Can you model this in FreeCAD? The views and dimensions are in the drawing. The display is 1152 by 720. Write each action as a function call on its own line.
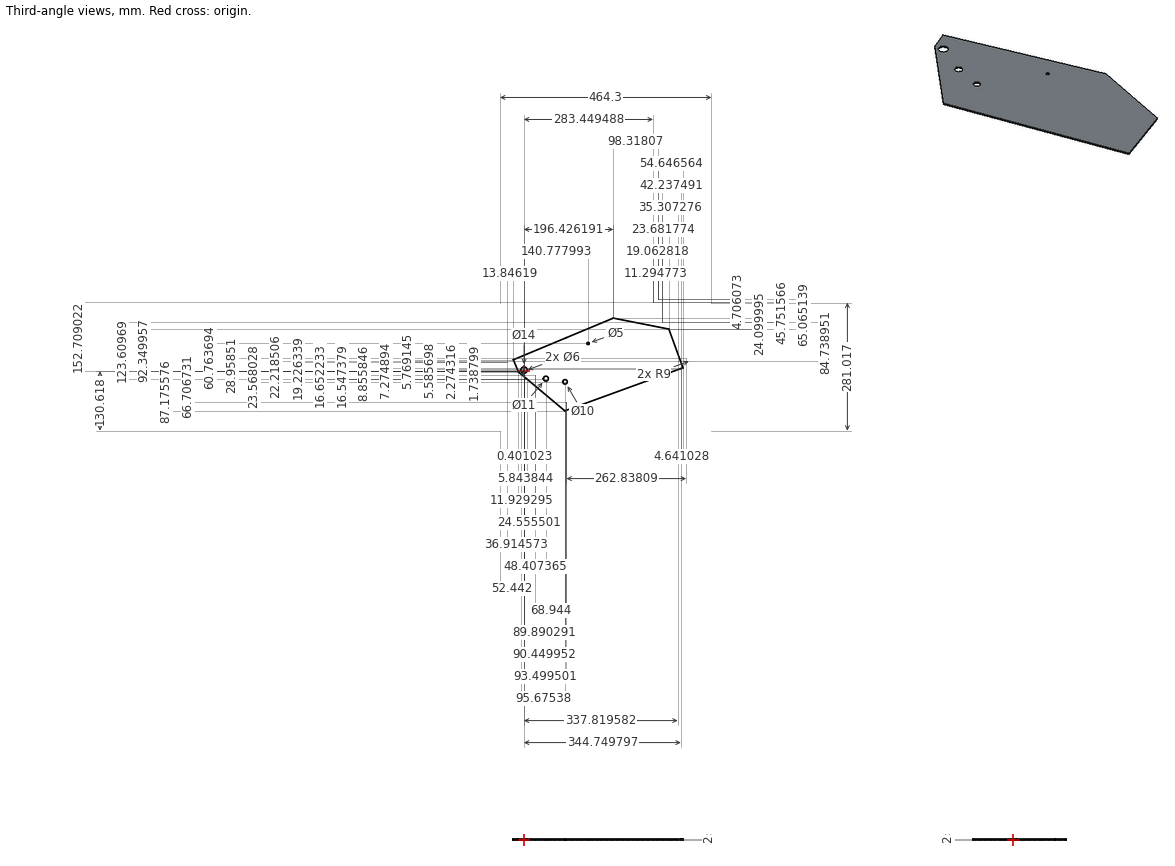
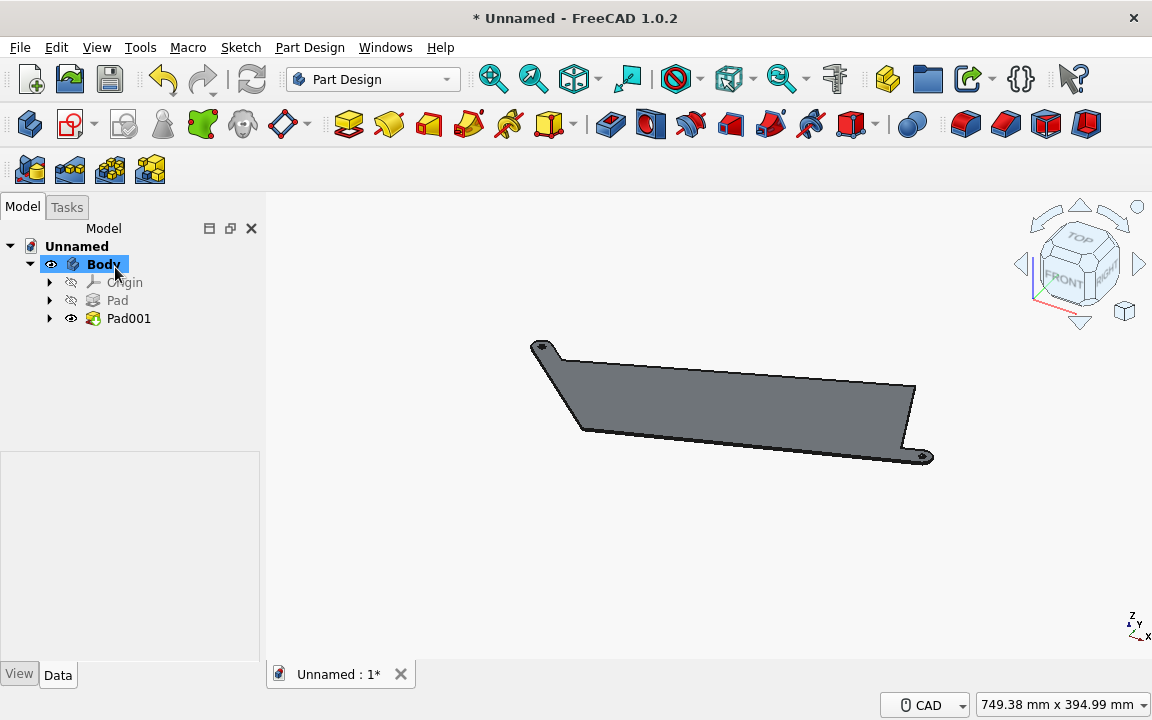
key(5)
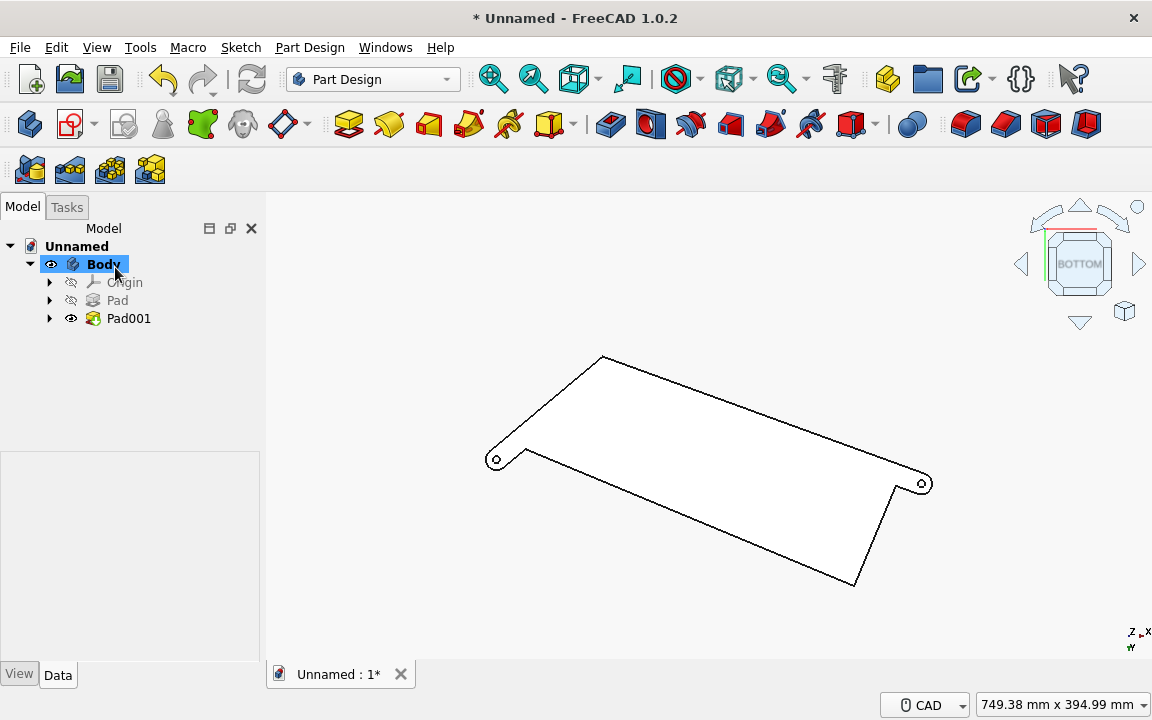
click(645, 438)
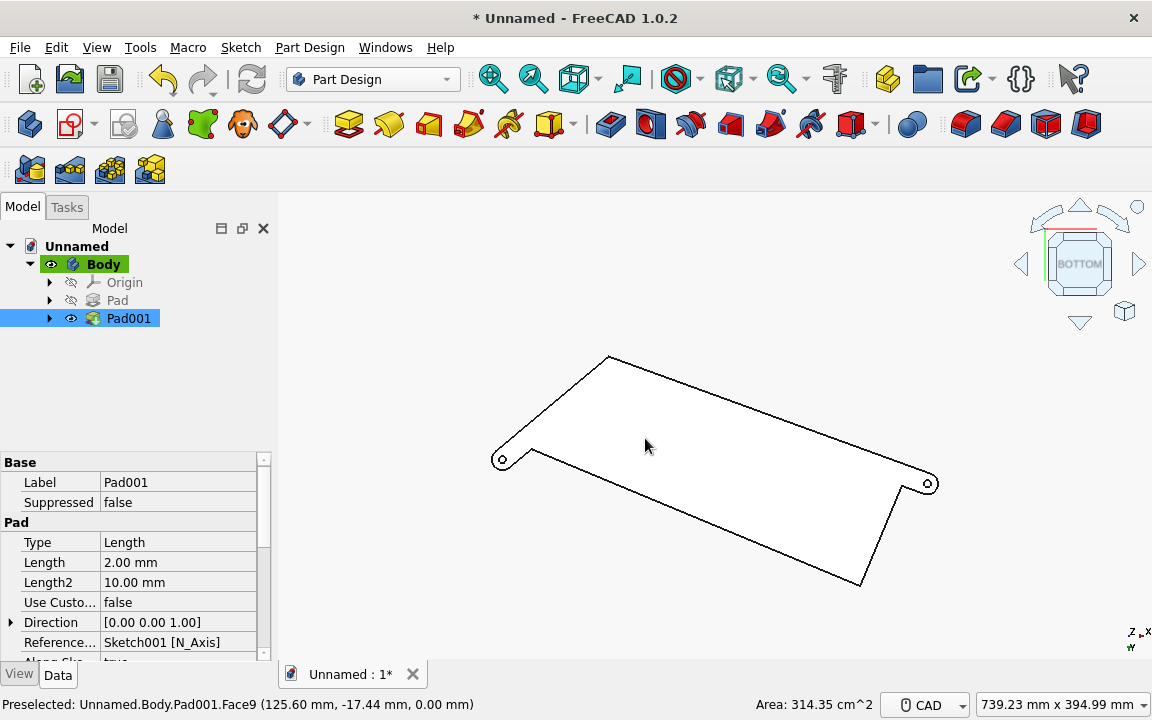
click(70, 124)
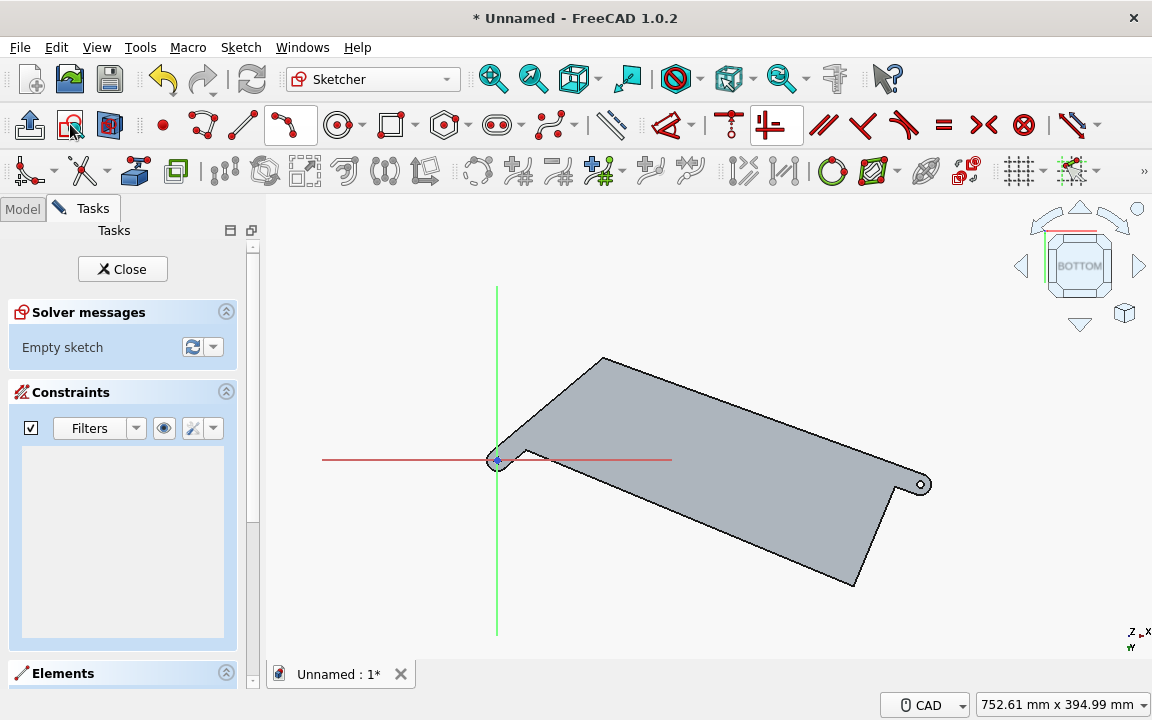
scroll(331, 222, down, 1)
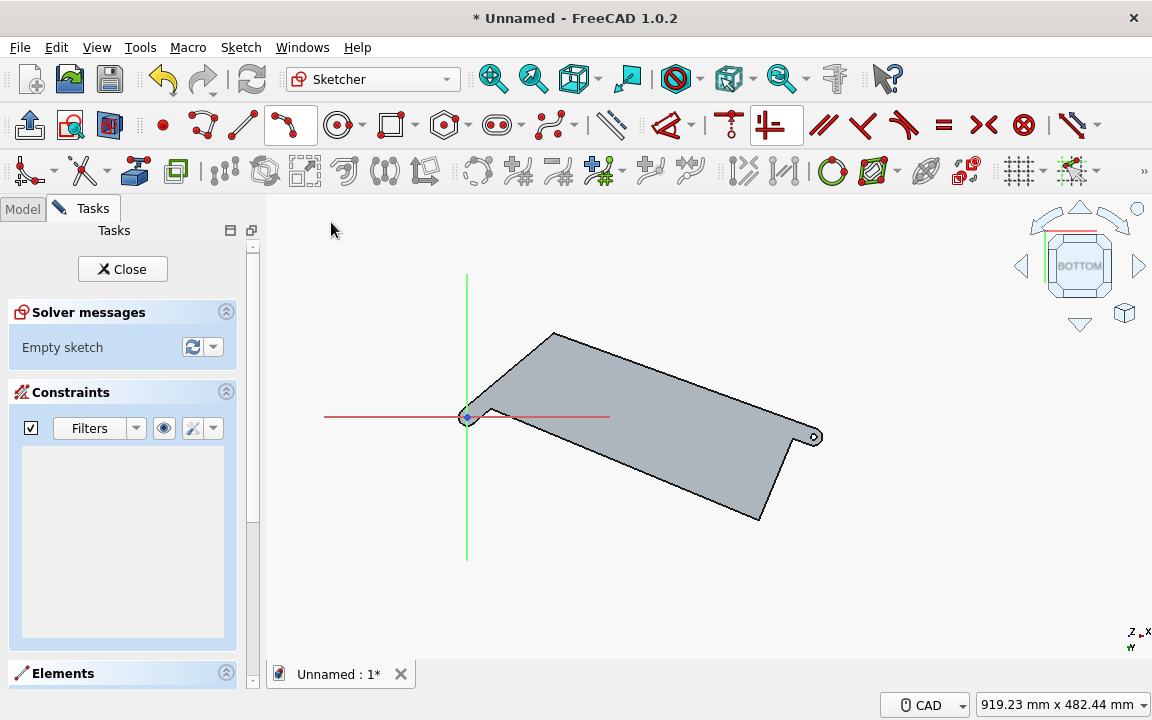
key(g)
key(r)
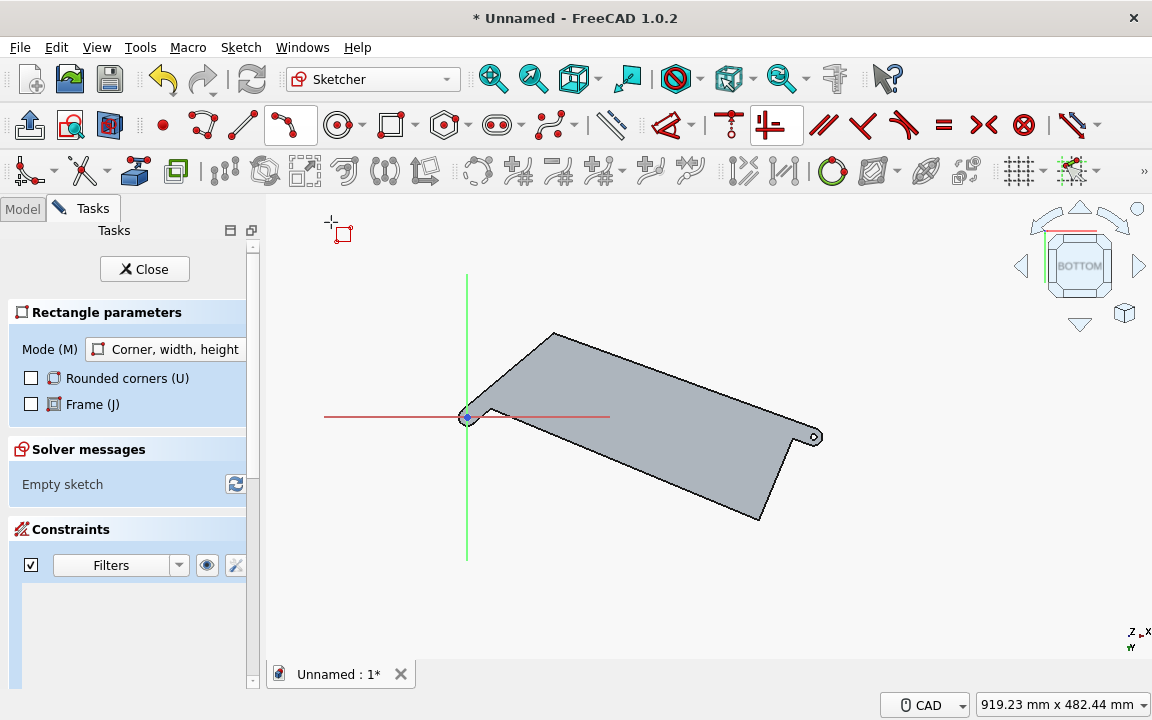
click(417, 291)
move(864, 562)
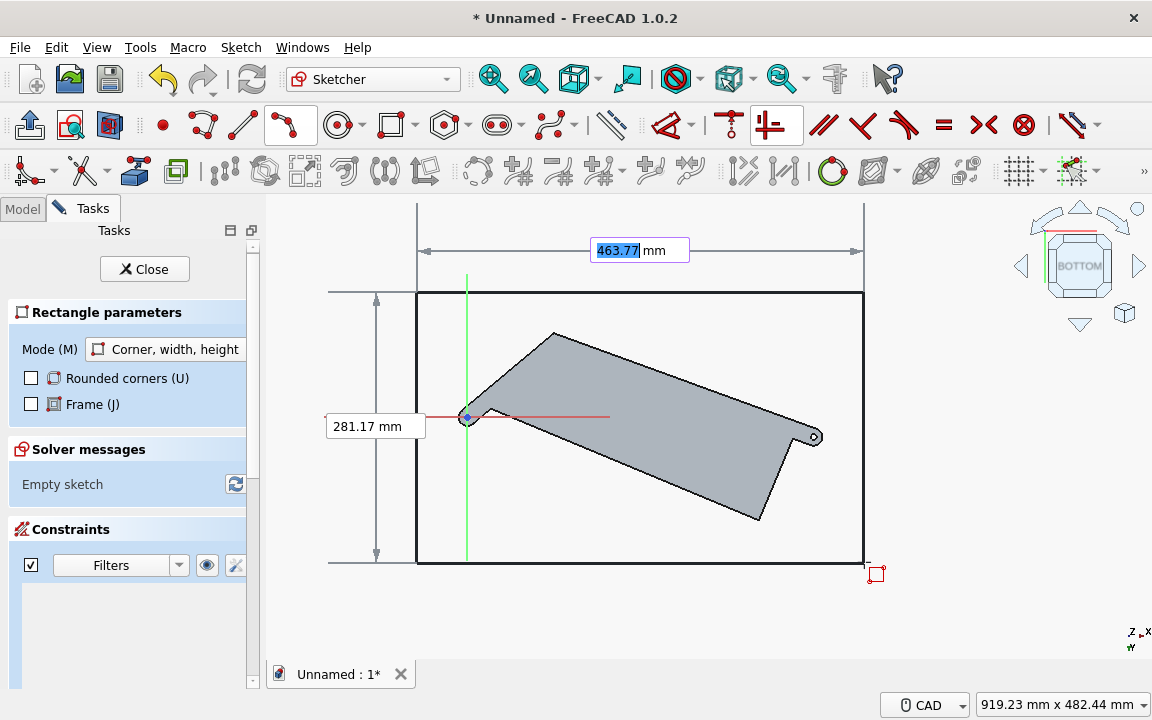
text(464.3)
key(Tab)
text(281.017)
key(Return)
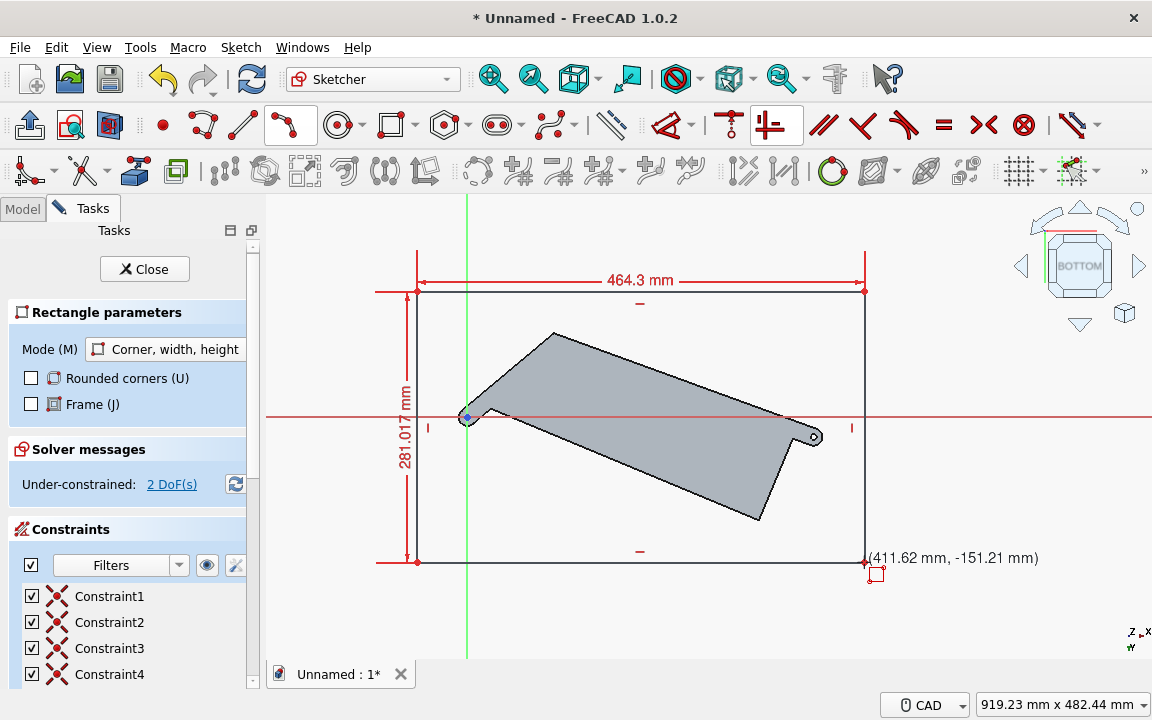
key(g)
key(m)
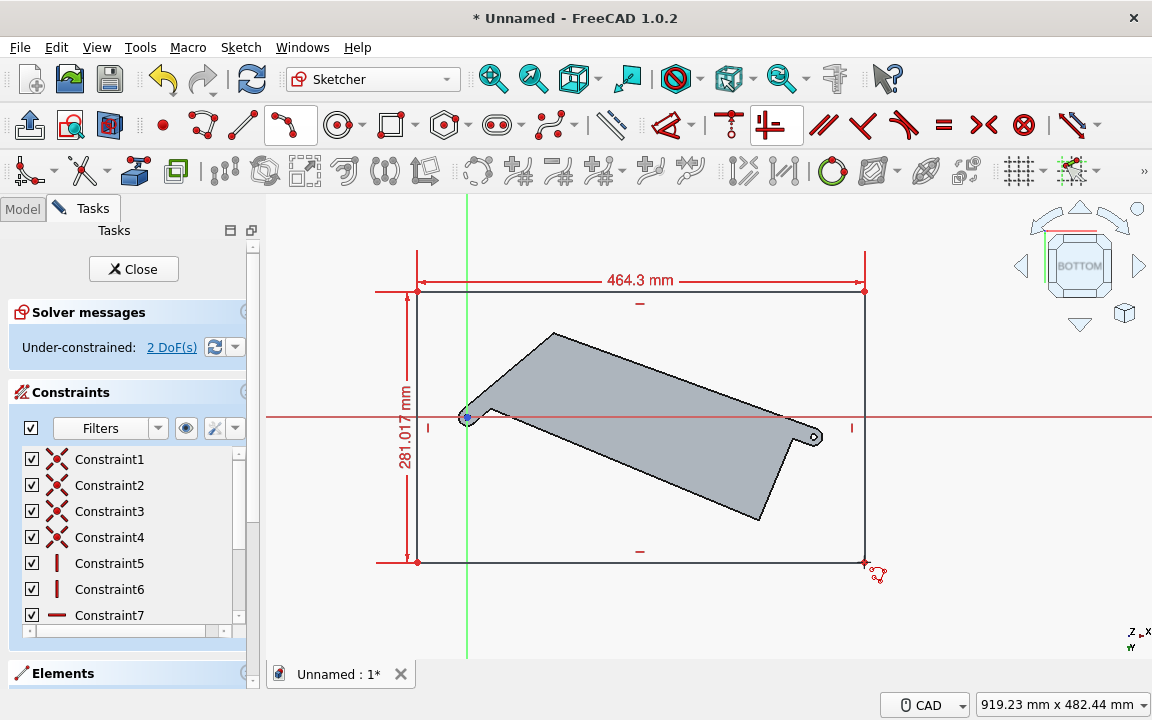
scroll(473, 401, up, 6)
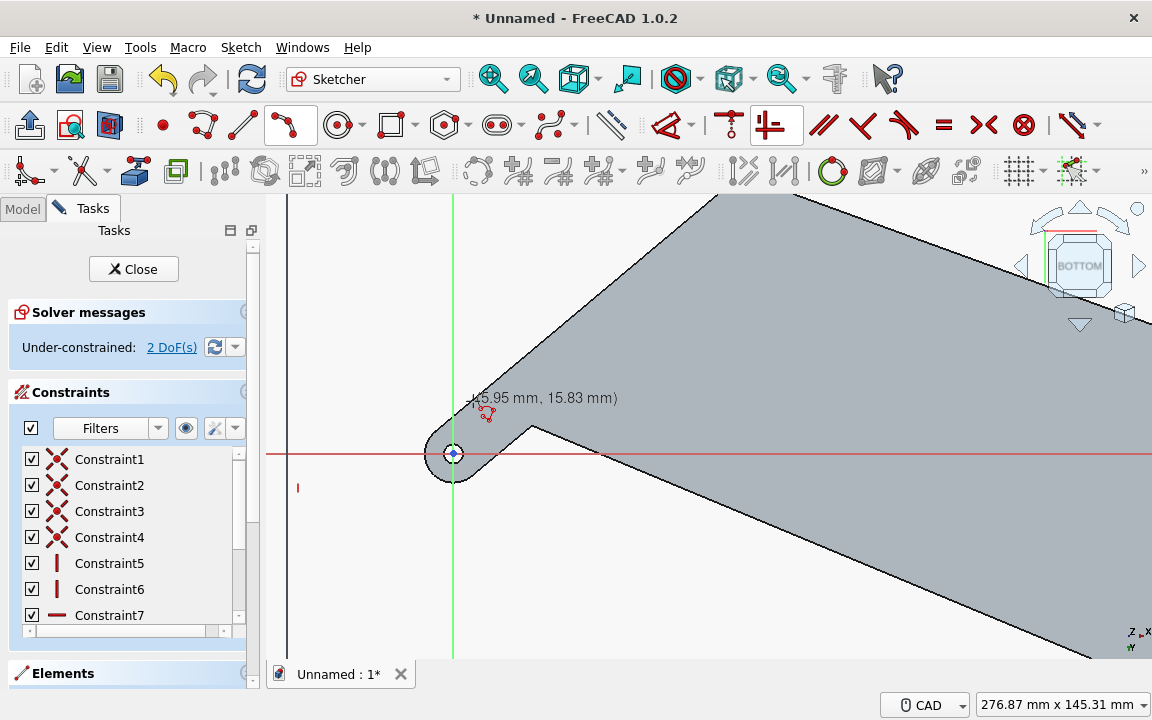
click(472, 401)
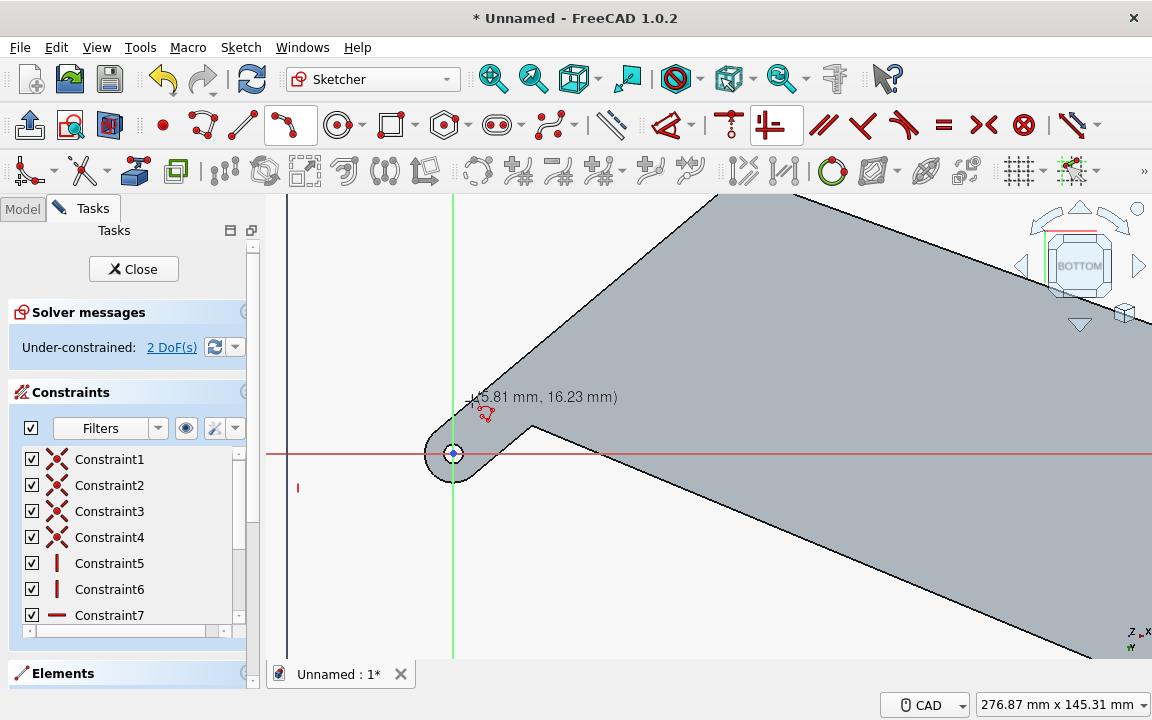
scroll(473, 401, down, 6)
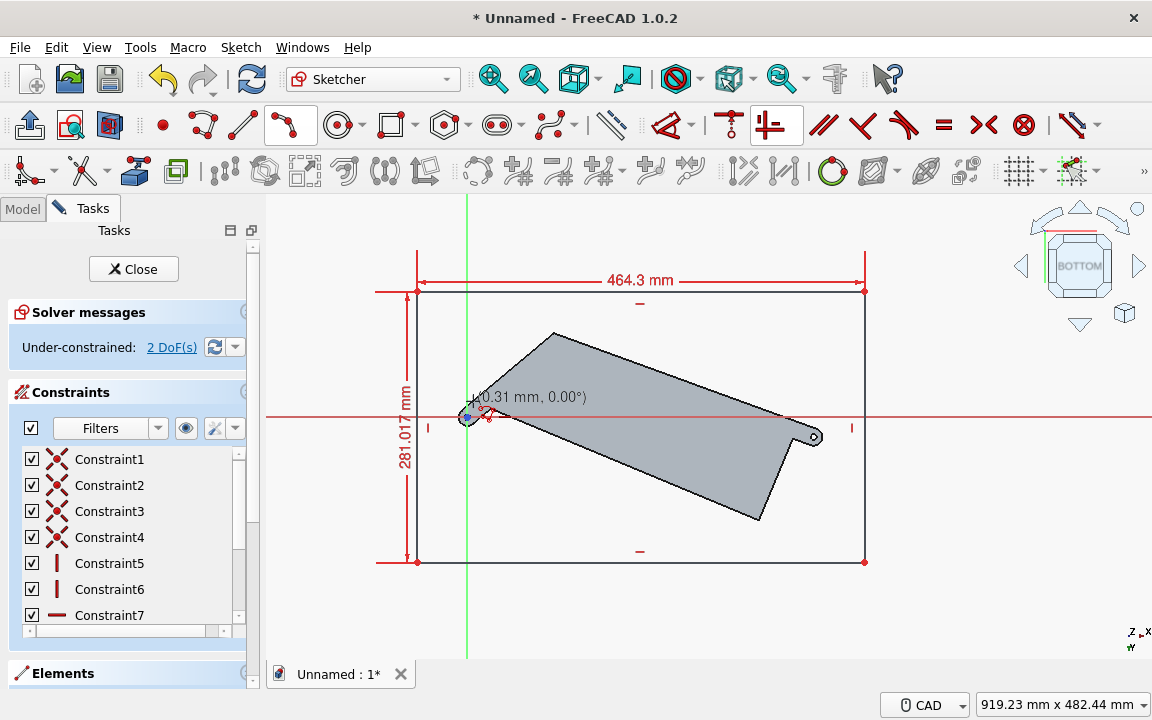
click(554, 333)